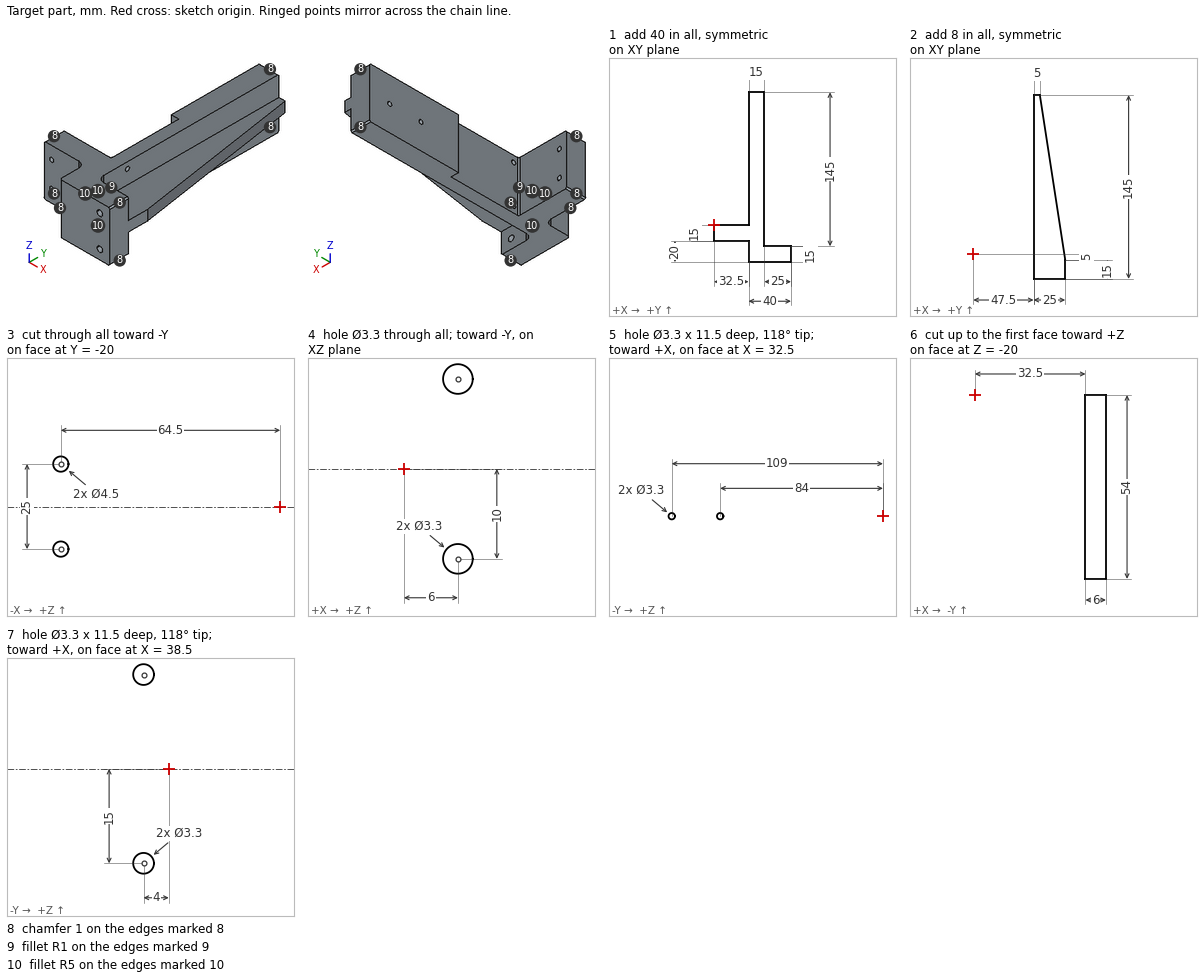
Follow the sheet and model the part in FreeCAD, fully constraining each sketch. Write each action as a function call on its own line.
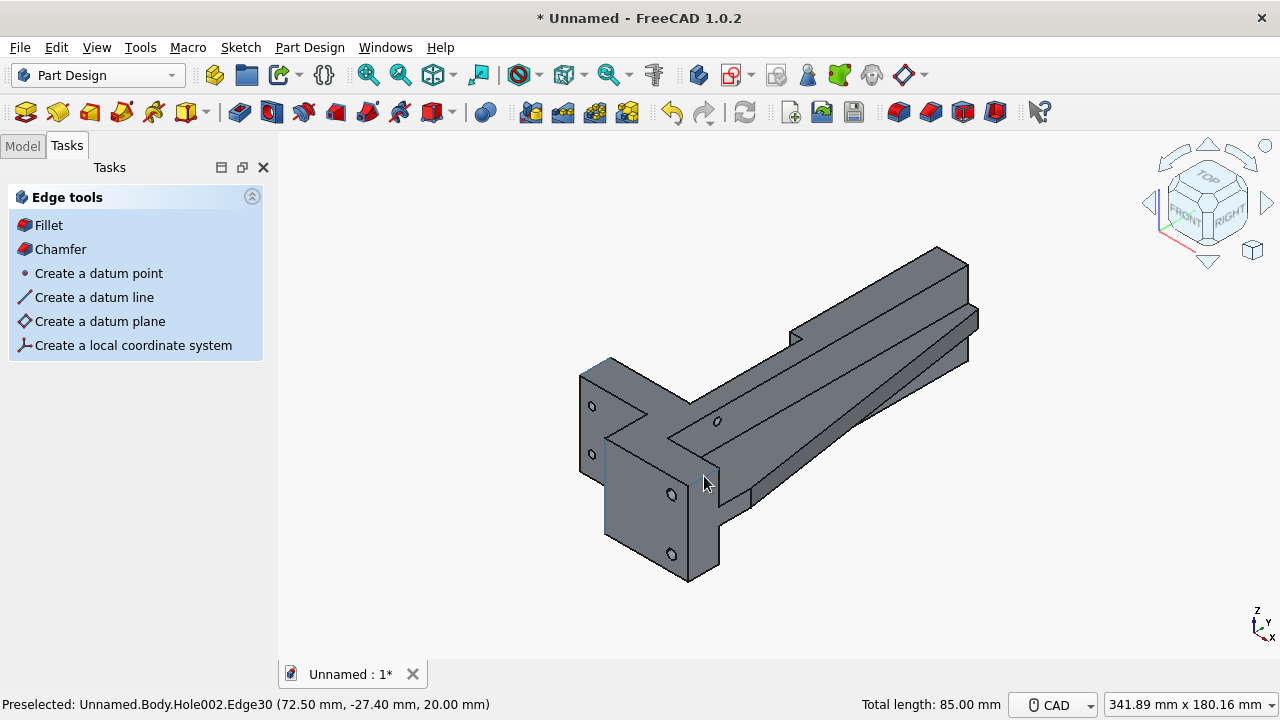
key(2)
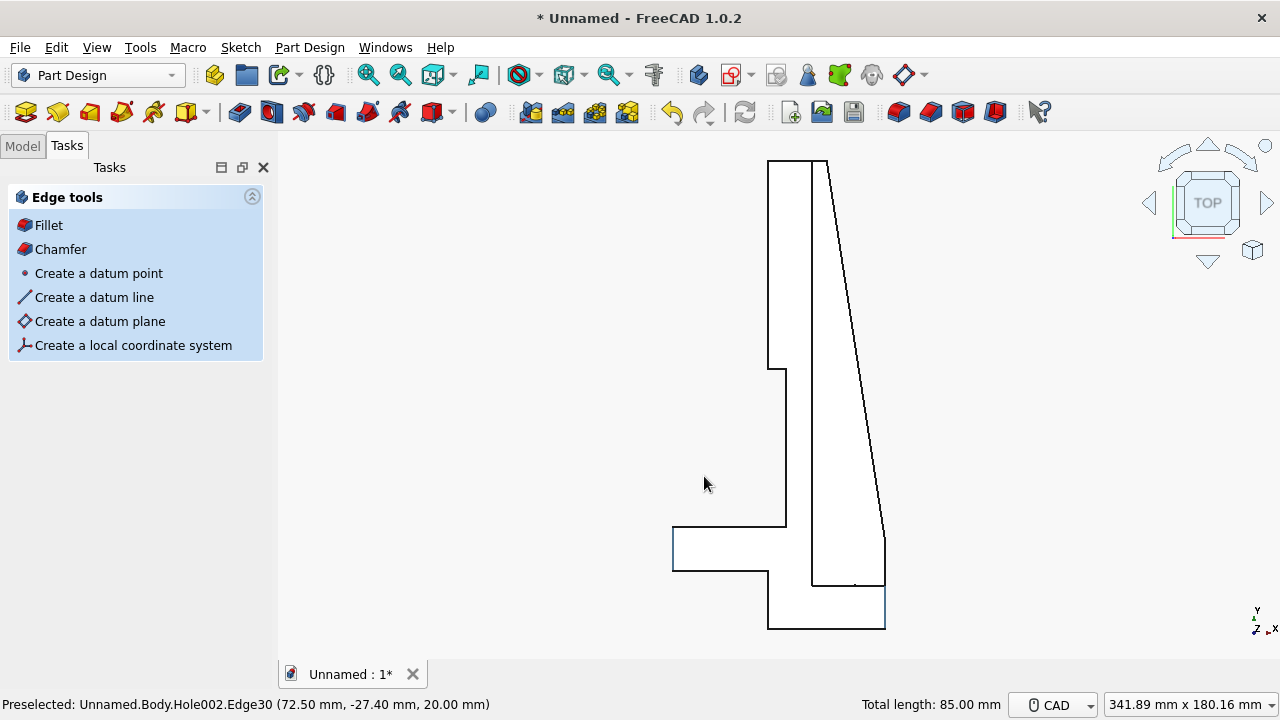
click(790, 160, ctrl)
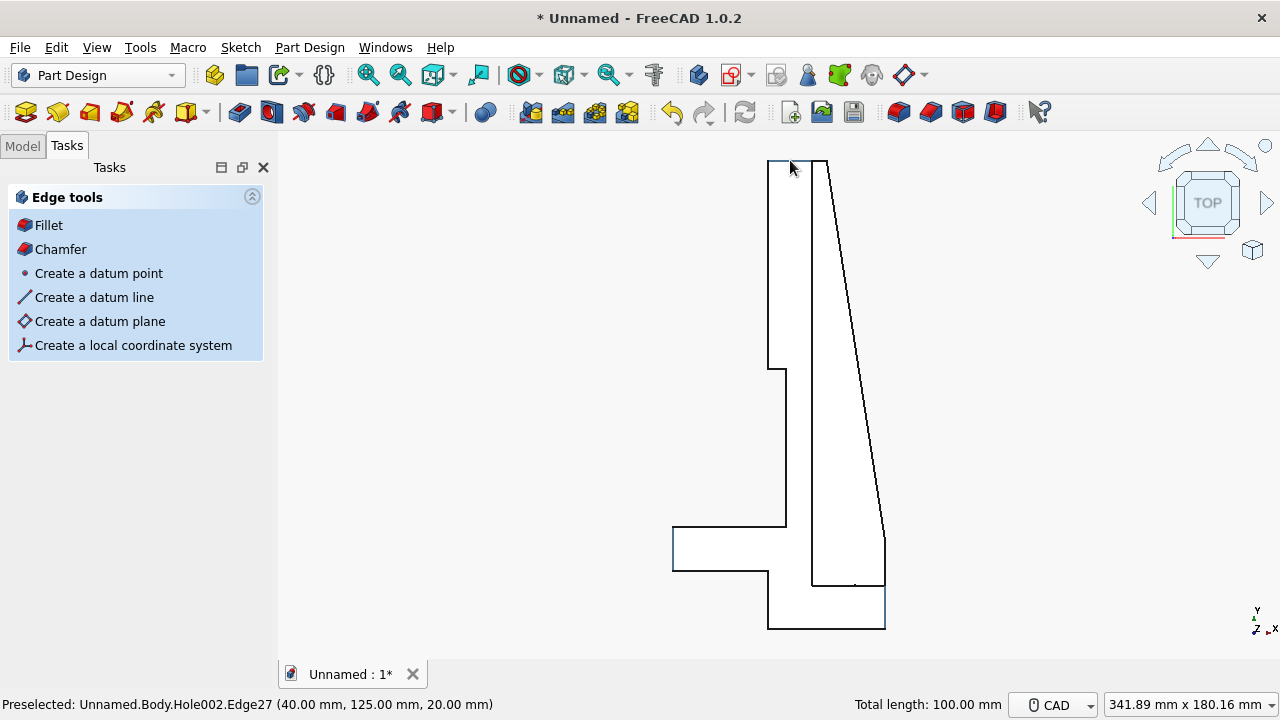
key(1)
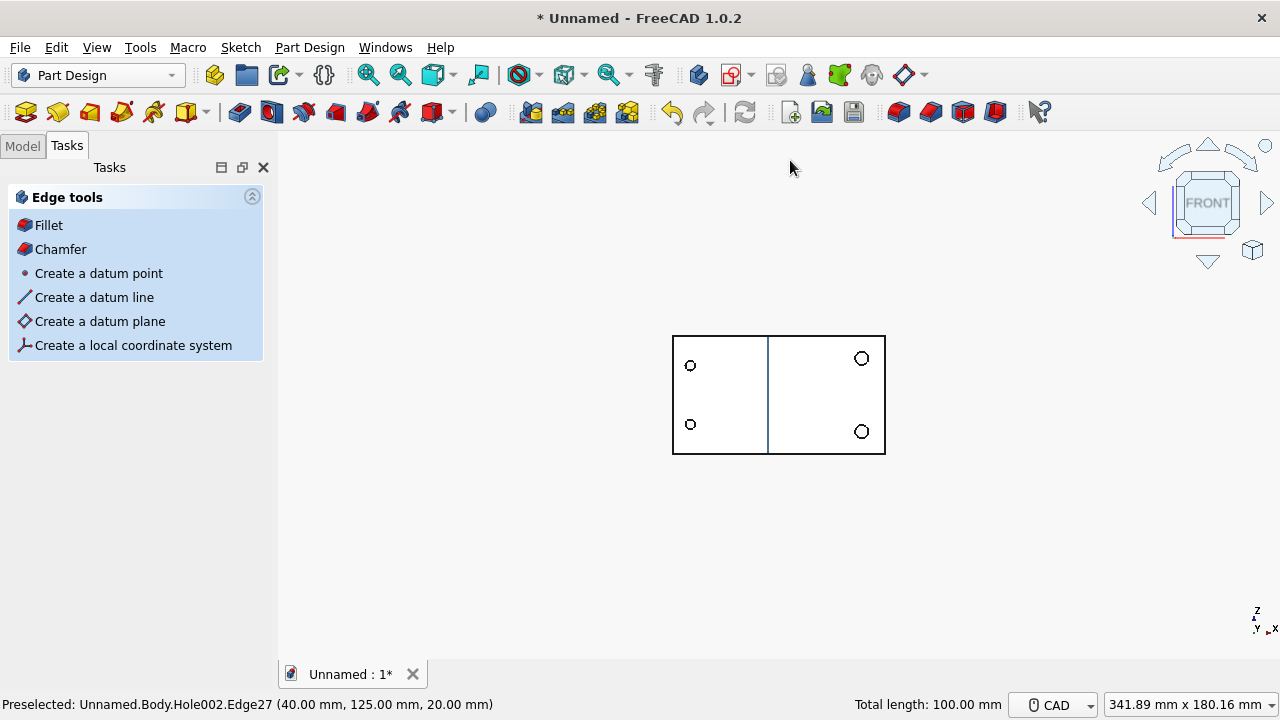
key(v)
key(f)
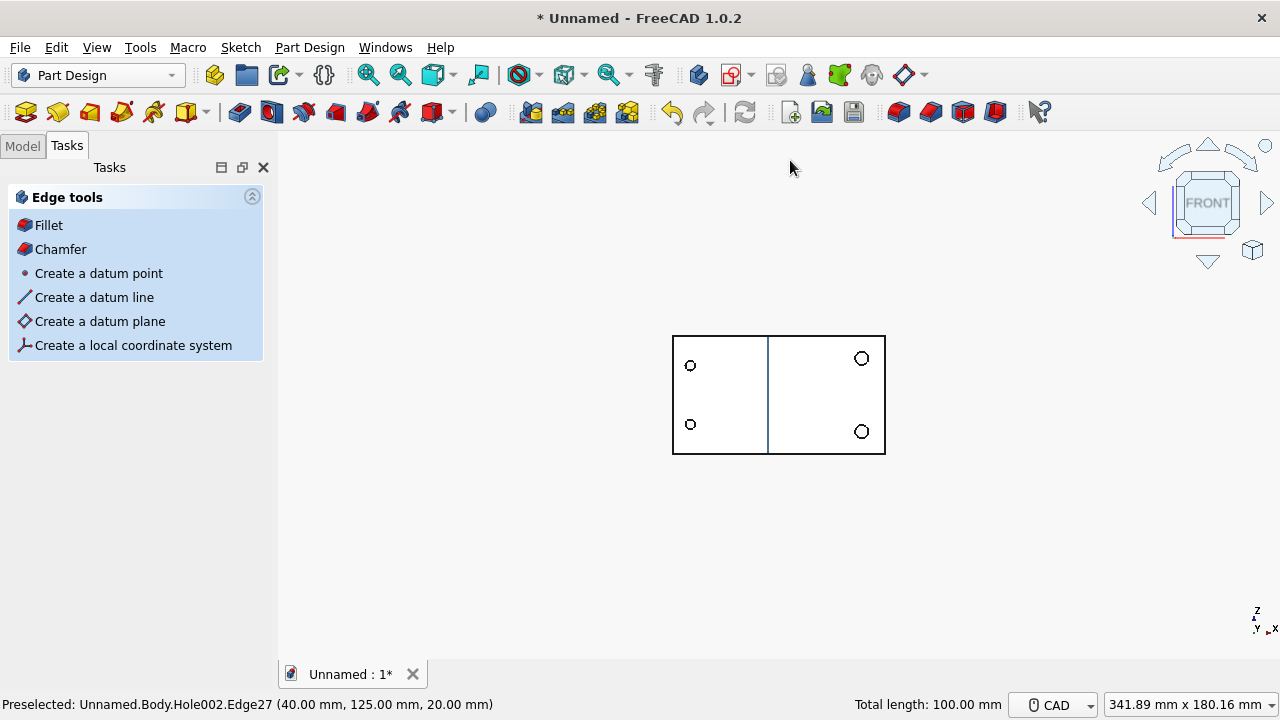
key(3)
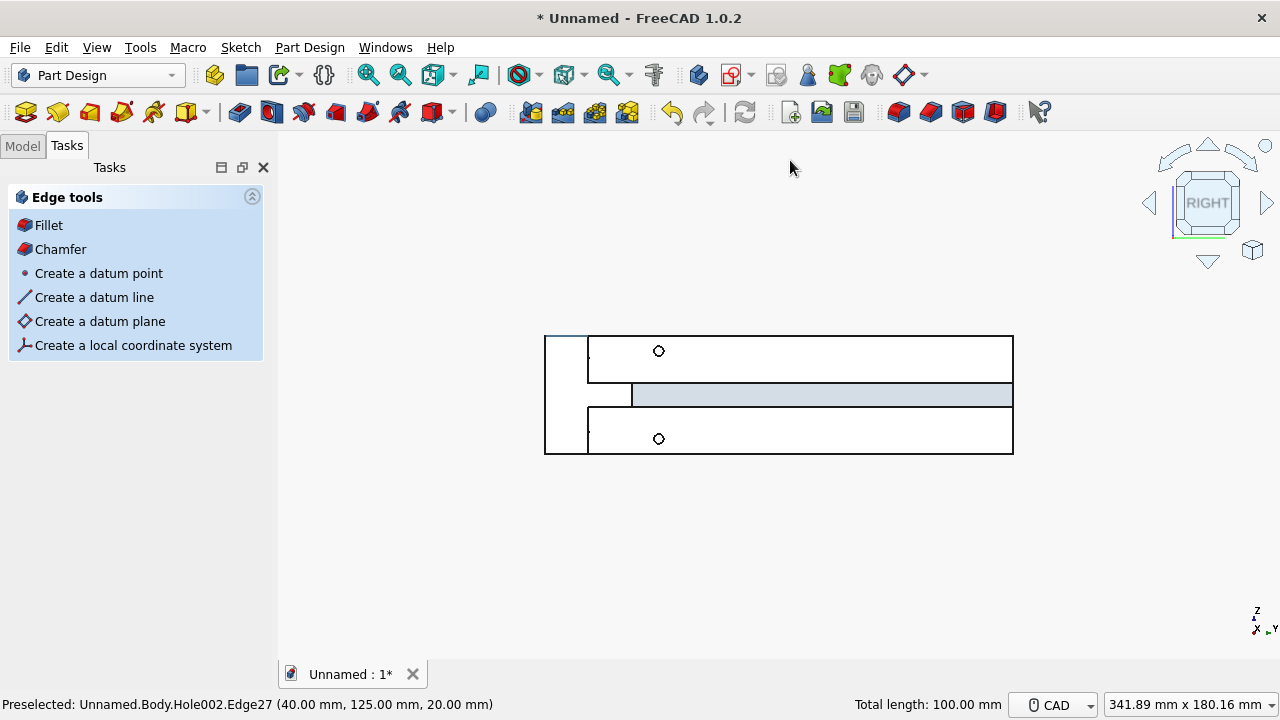
click(567, 453, ctrl)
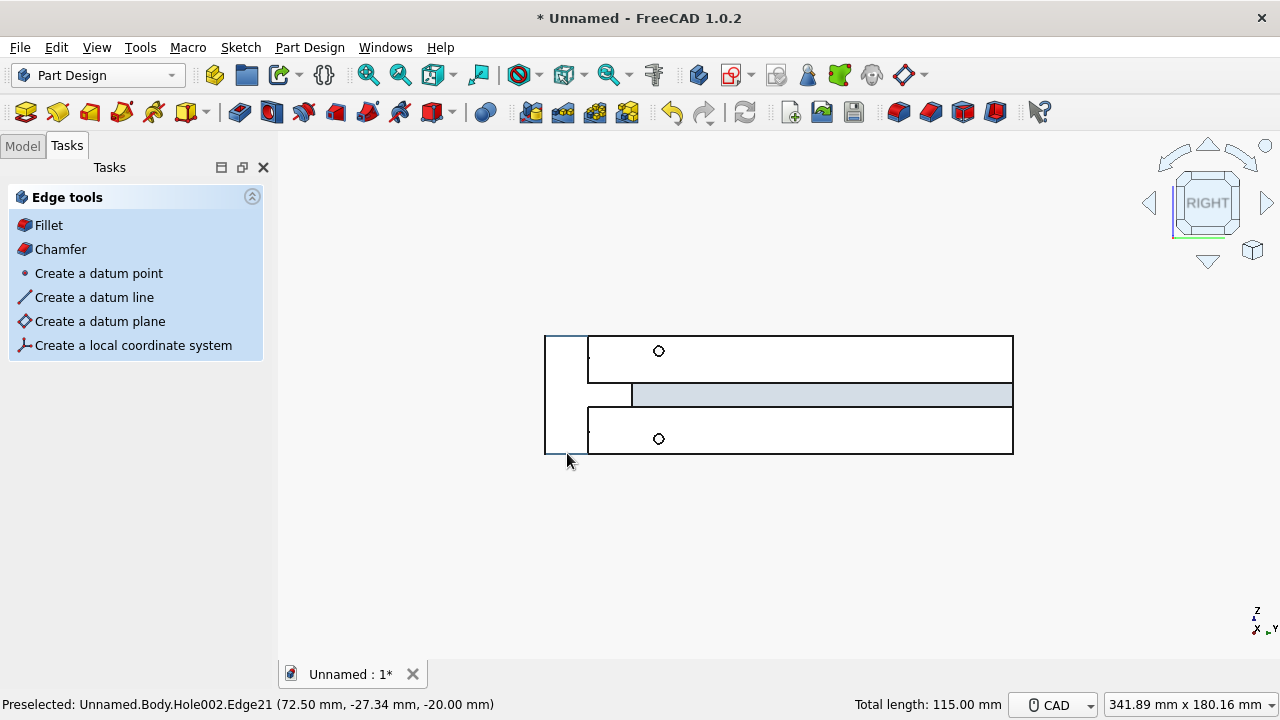
key(5)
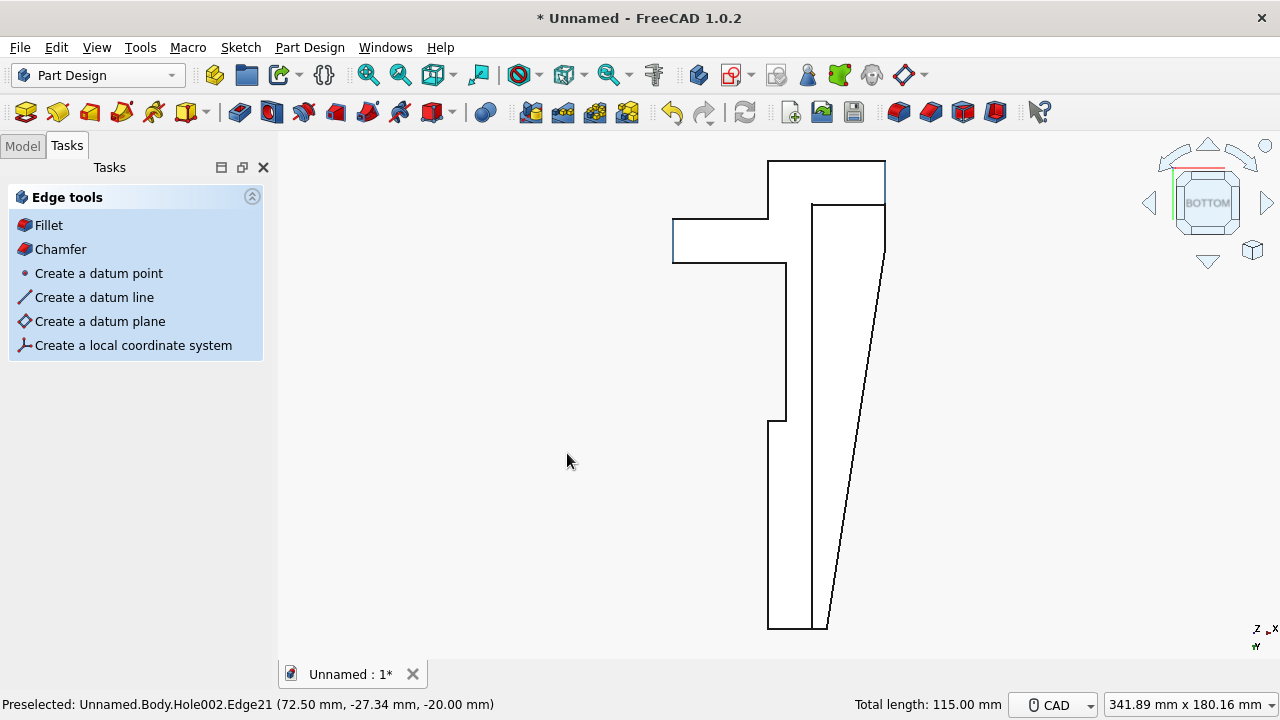
click(790, 628, ctrl)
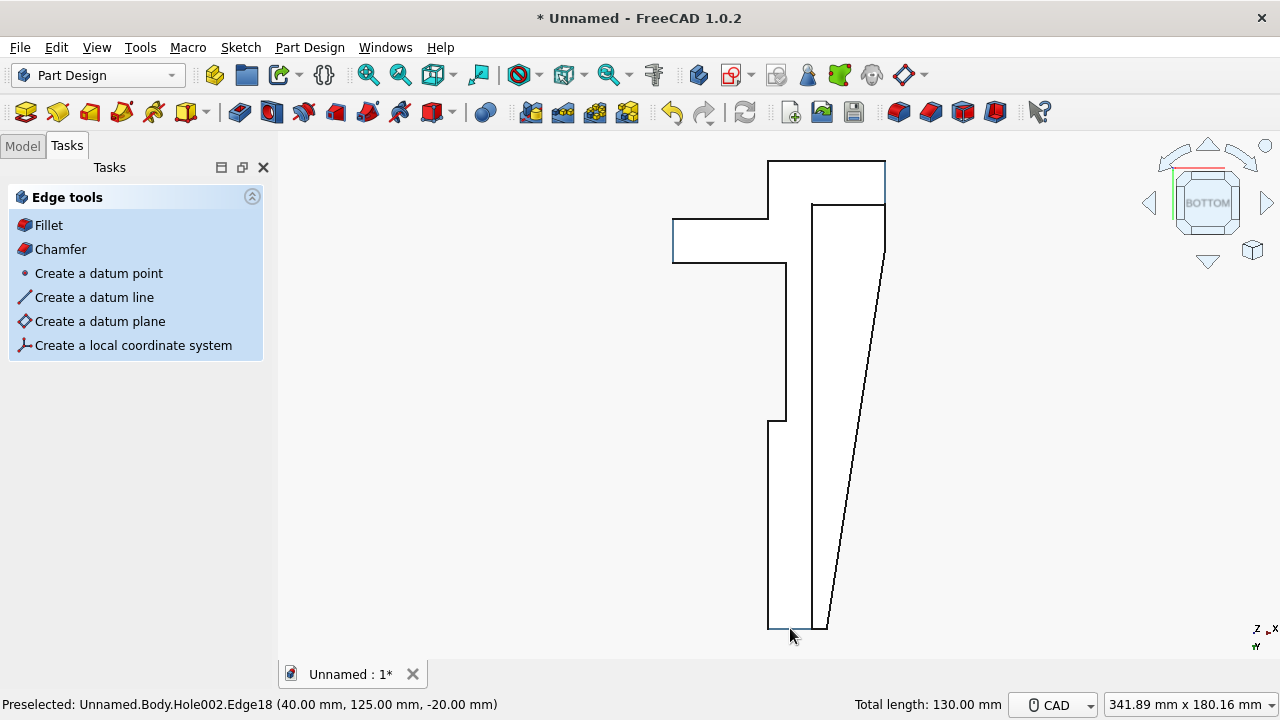
click(932, 112)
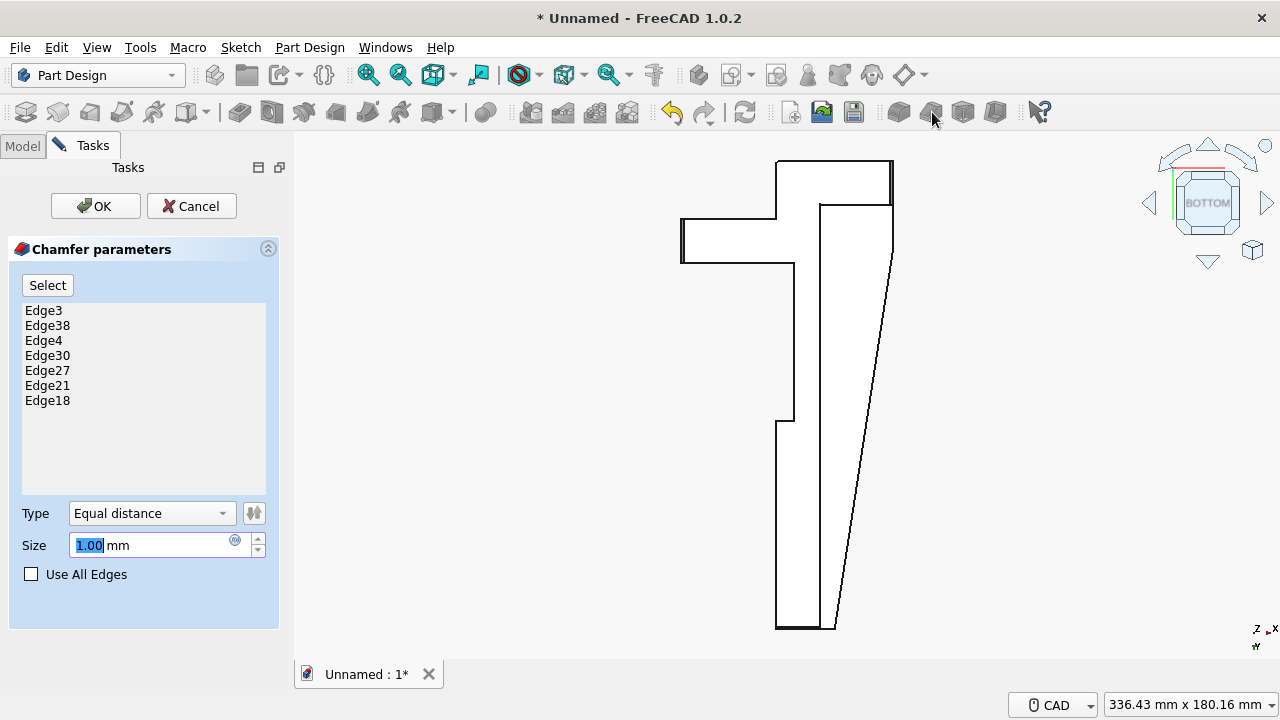
text(1)
key(Tab)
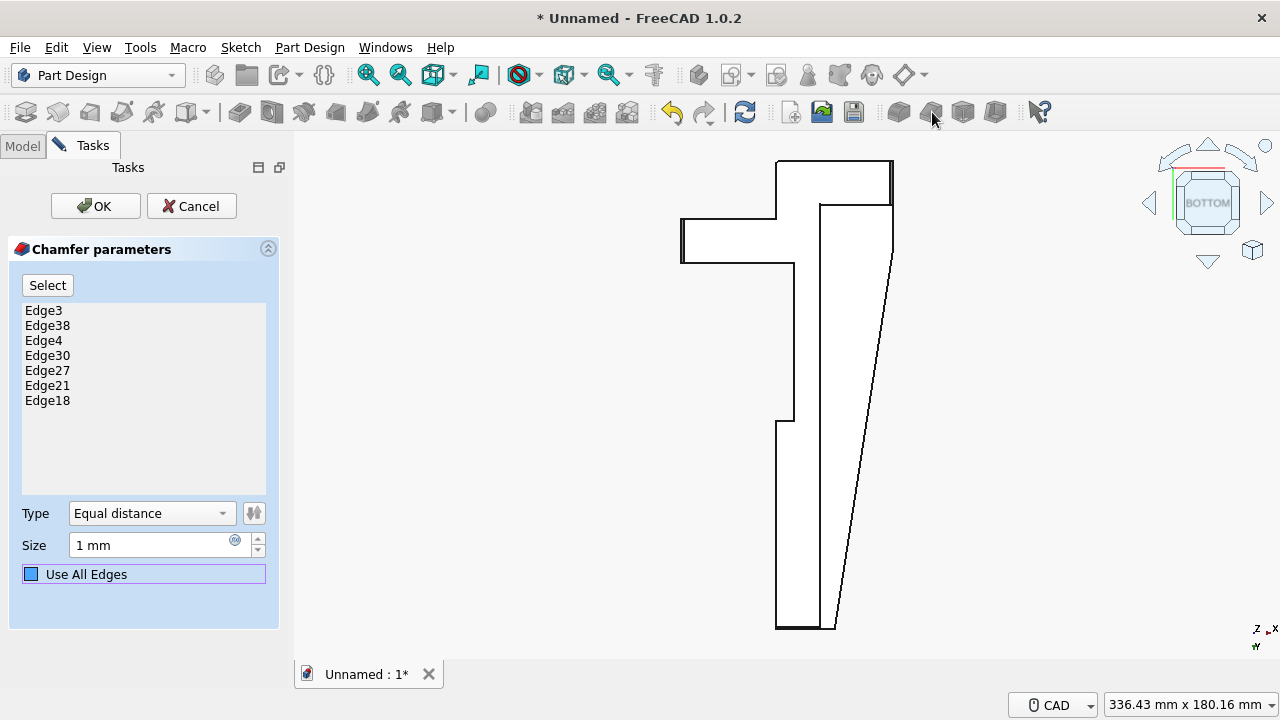
click(96, 206)